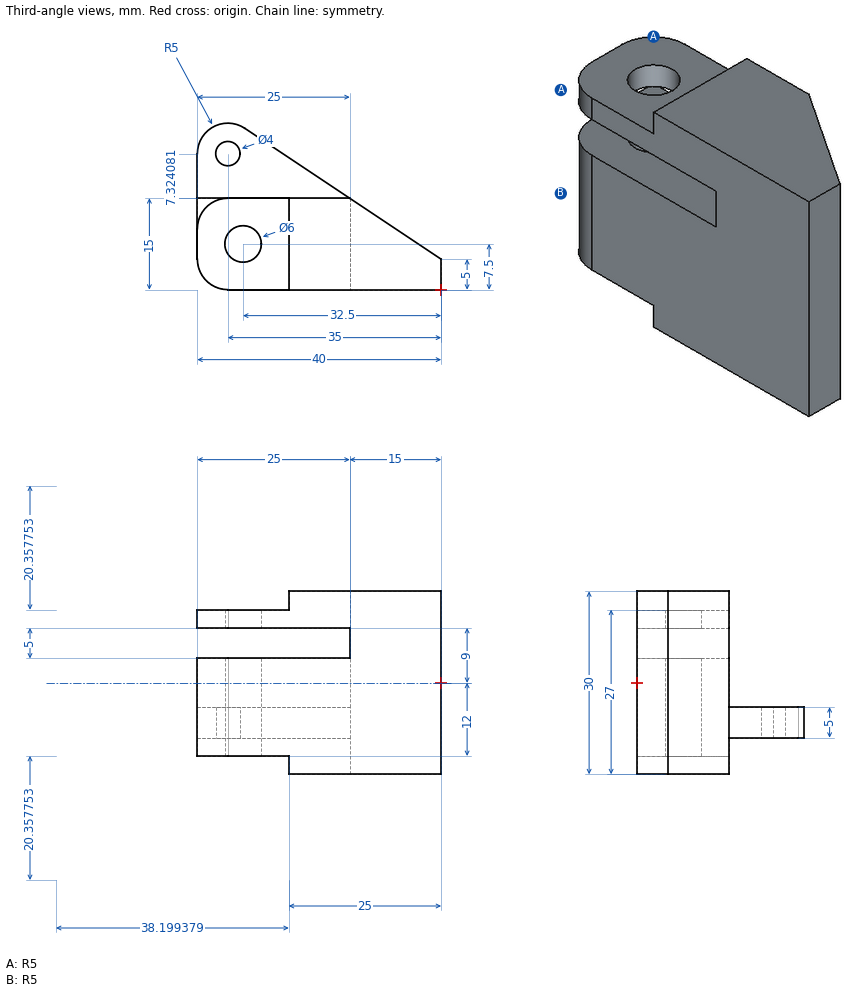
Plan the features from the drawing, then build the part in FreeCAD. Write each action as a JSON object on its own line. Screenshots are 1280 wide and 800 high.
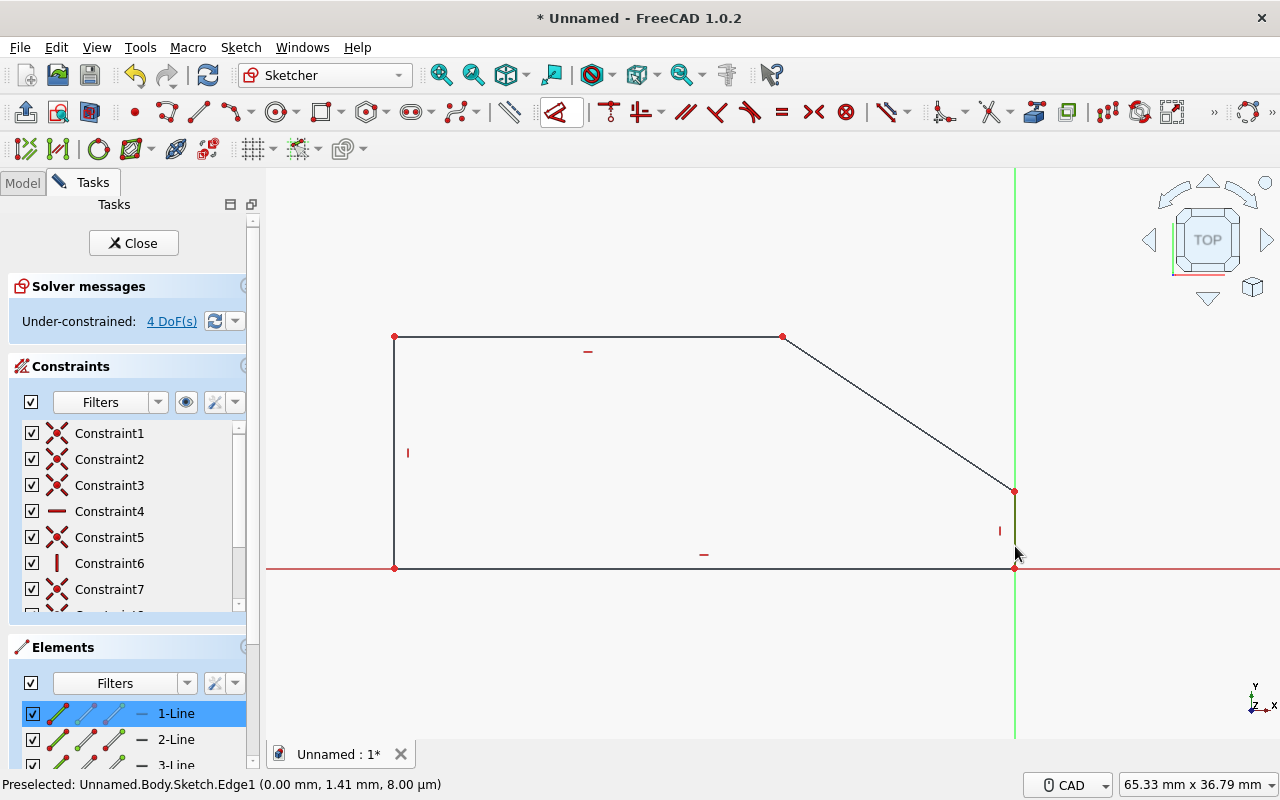
{"action": "key", "text": "i"}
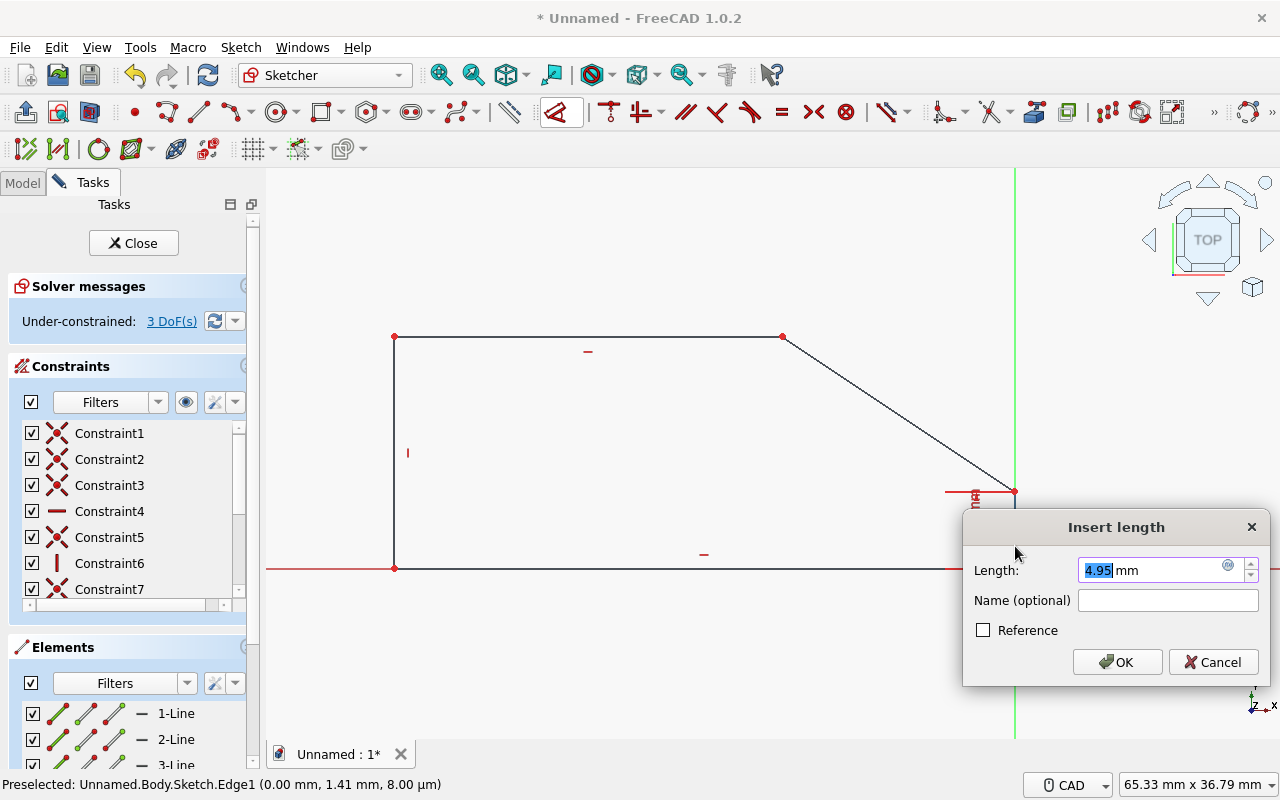
{"action": "type", "text": "5"}
{"action": "key", "text": "Return"}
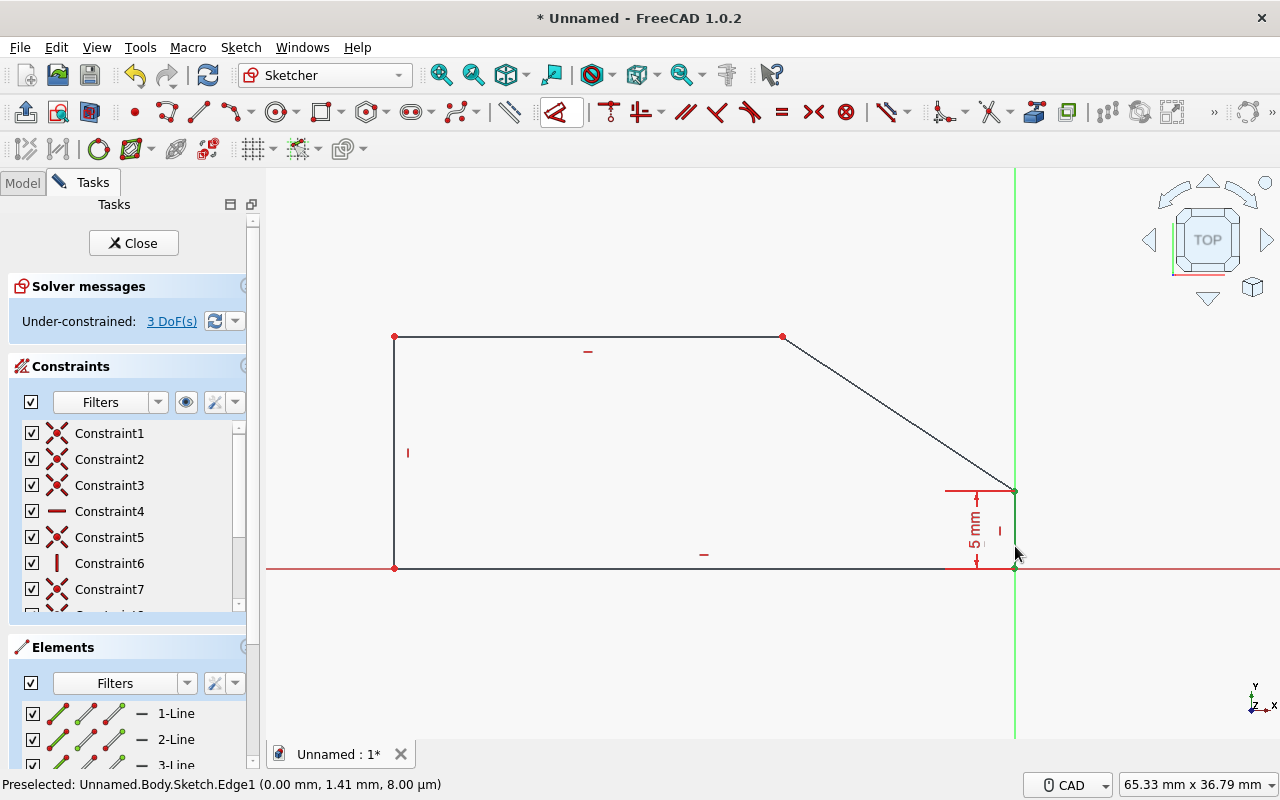
{"action": "left_click", "coordinate": [666, 337]}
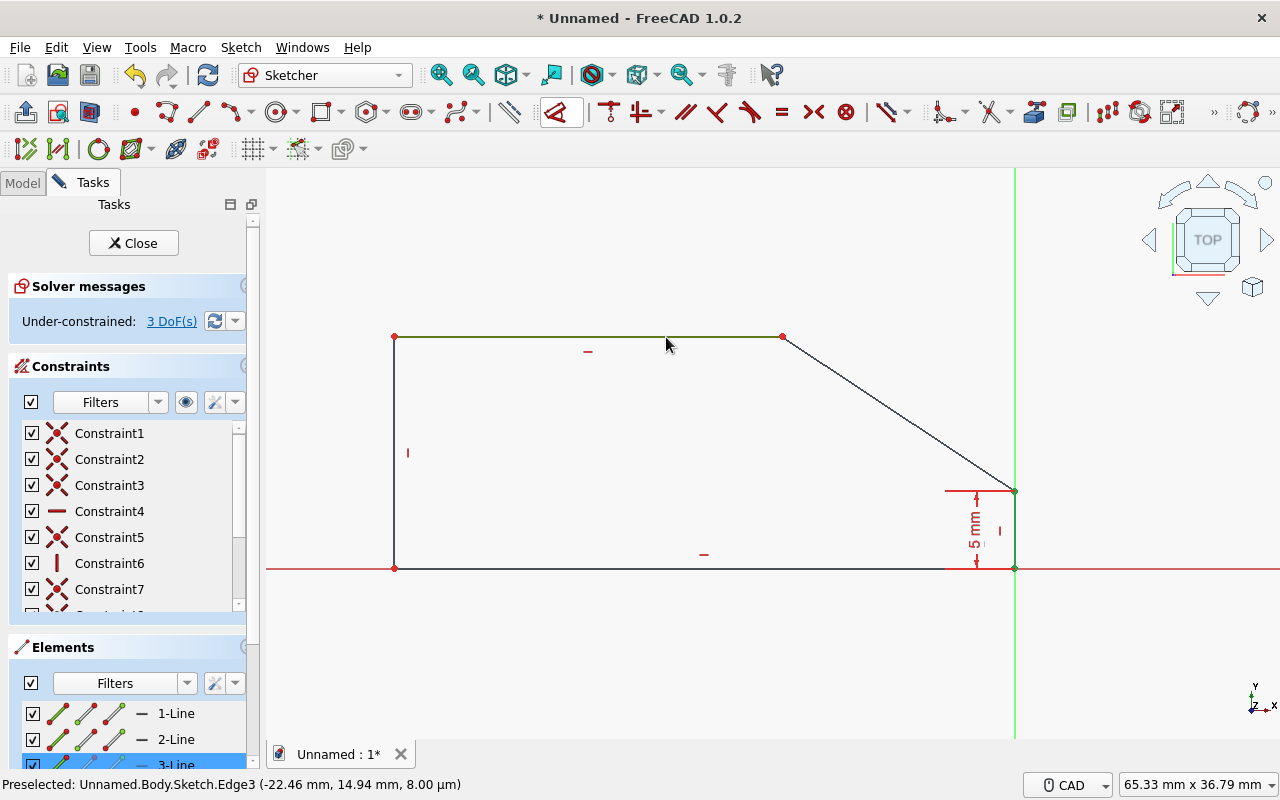
{"action": "key", "text": "l"}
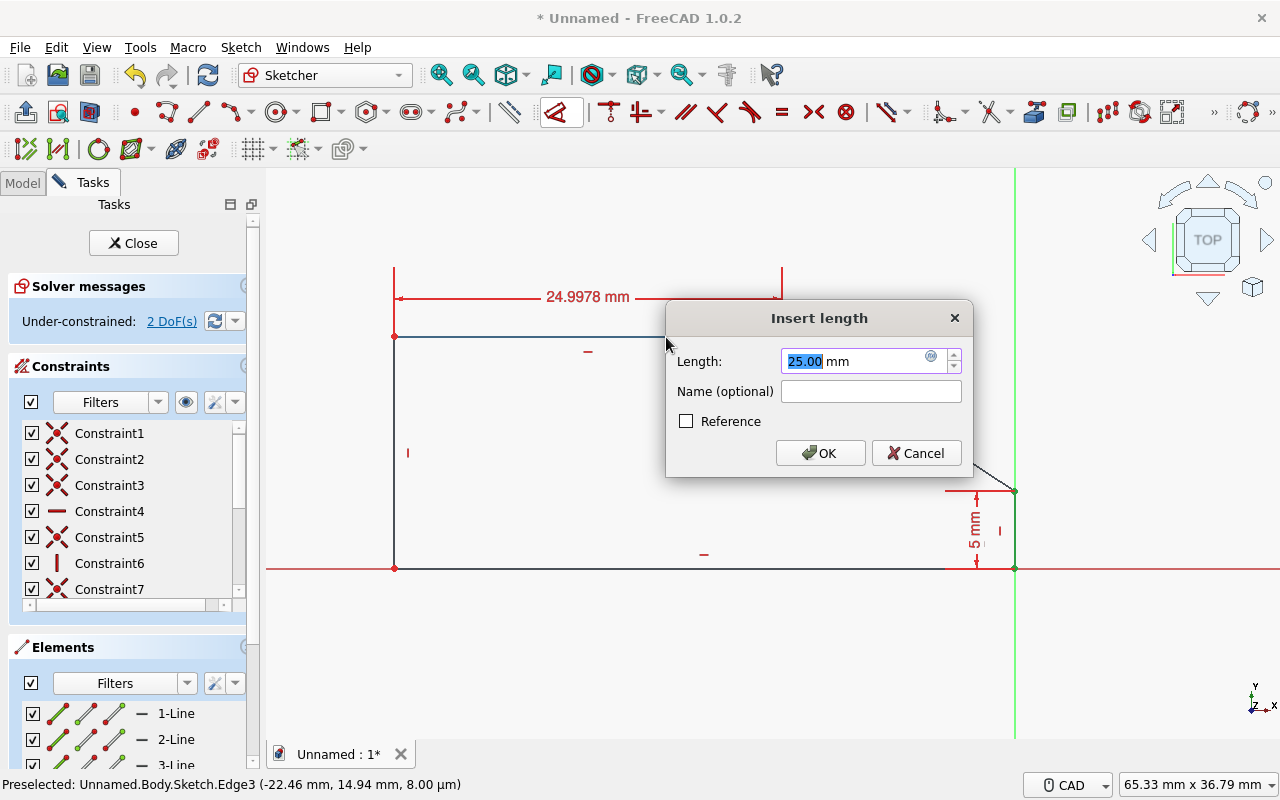
{"action": "type", "text": "25"}
{"action": "key", "text": "Return"}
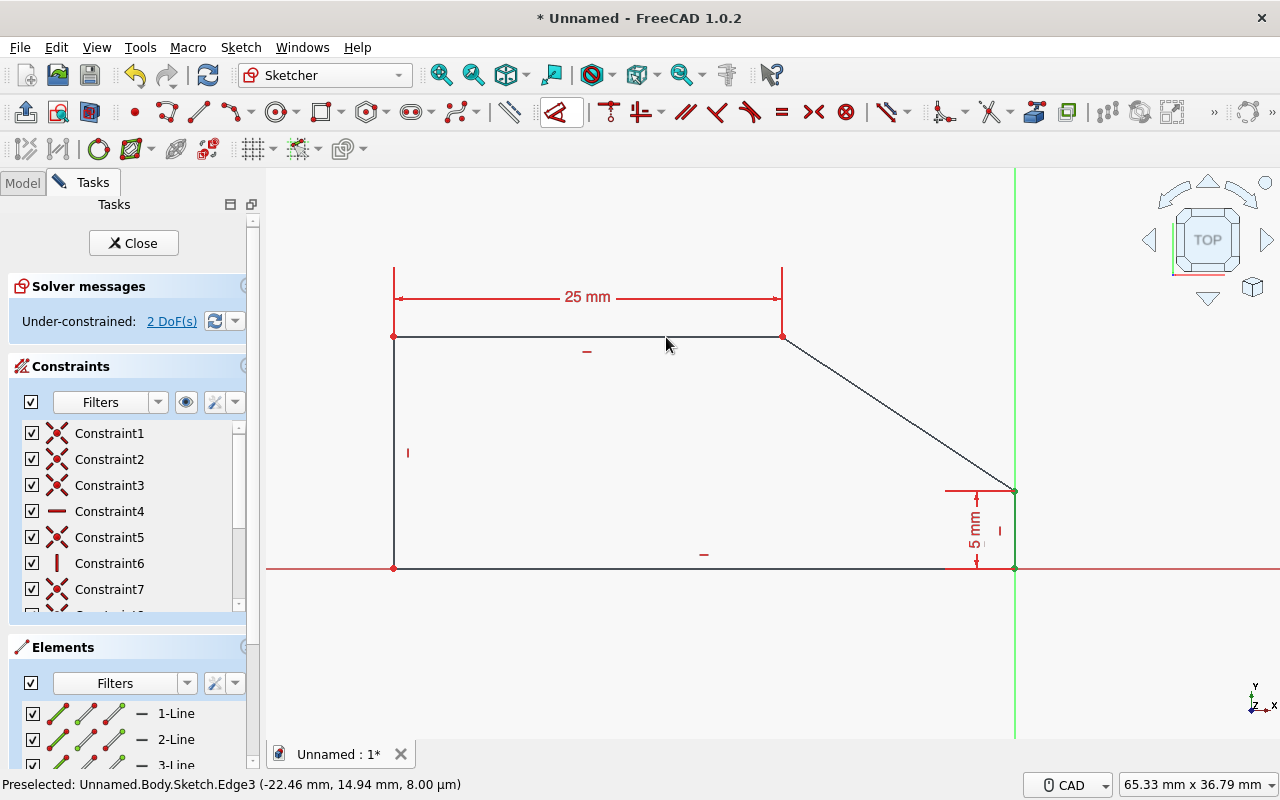
{"action": "left_click", "coordinate": [394, 407]}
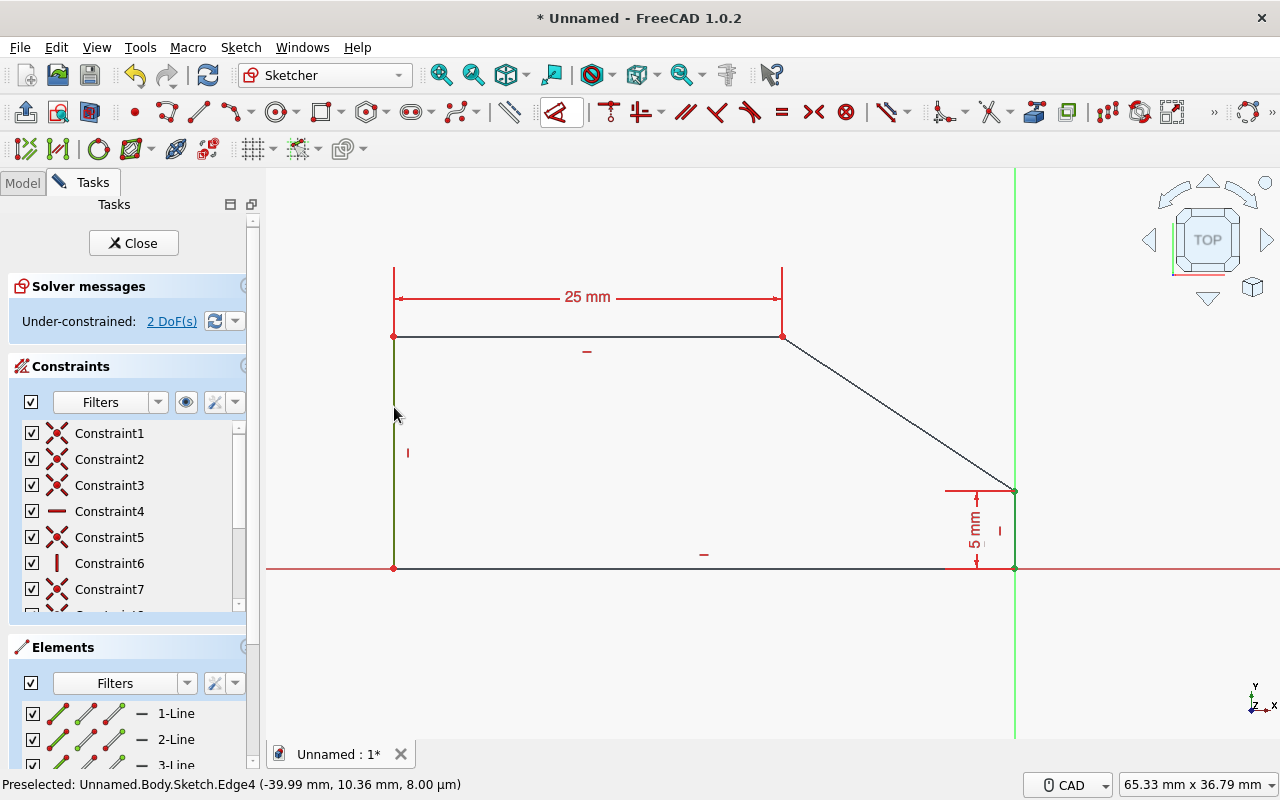
{"action": "left_click", "coordinate": [578, 112]}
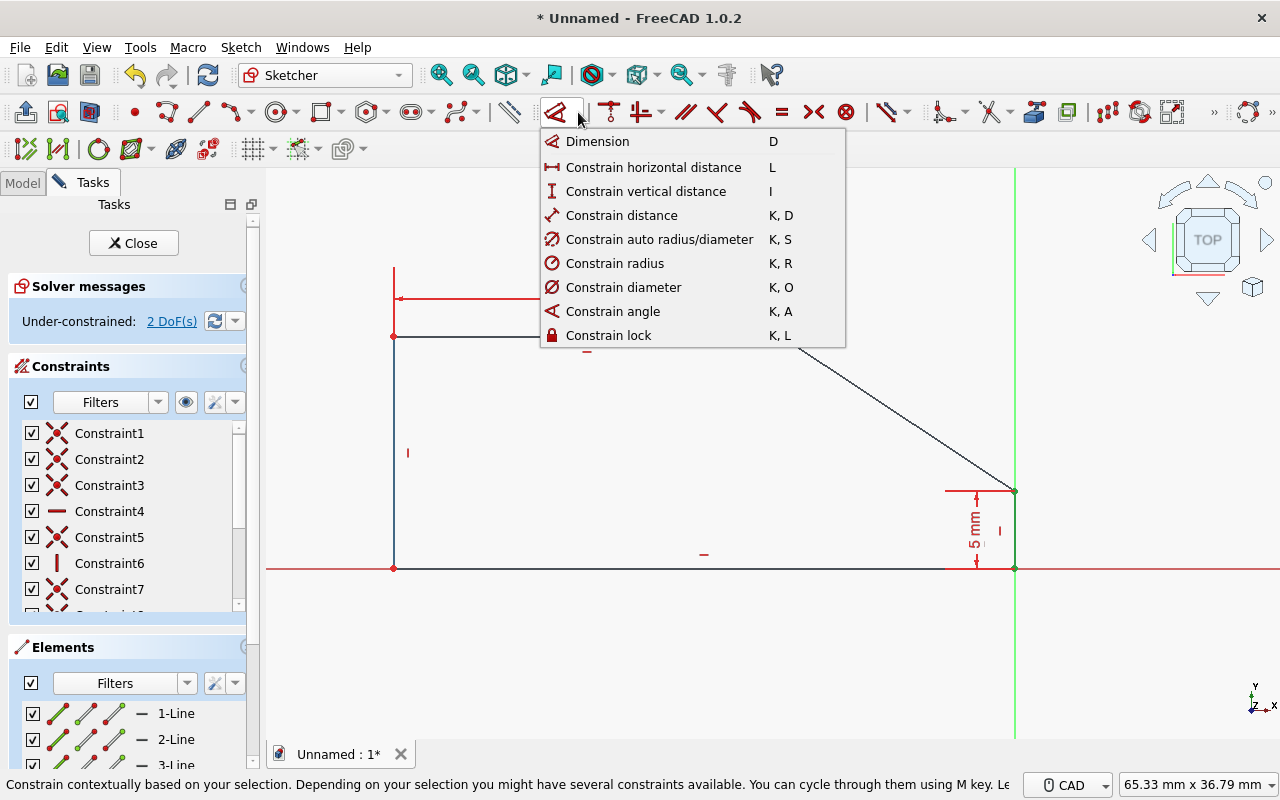
{"action": "left_click", "coordinate": [693, 191]}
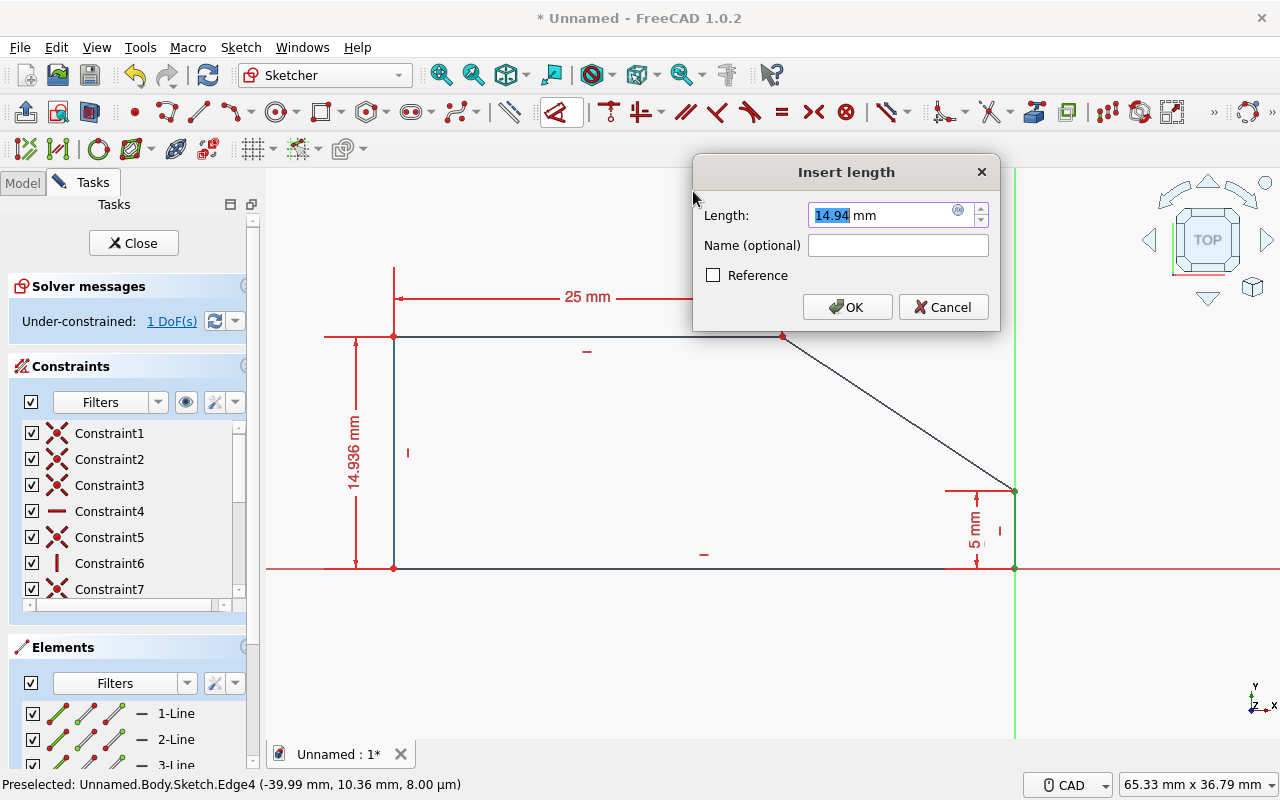
{"action": "type", "text": "15"}
{"action": "key", "text": "Return"}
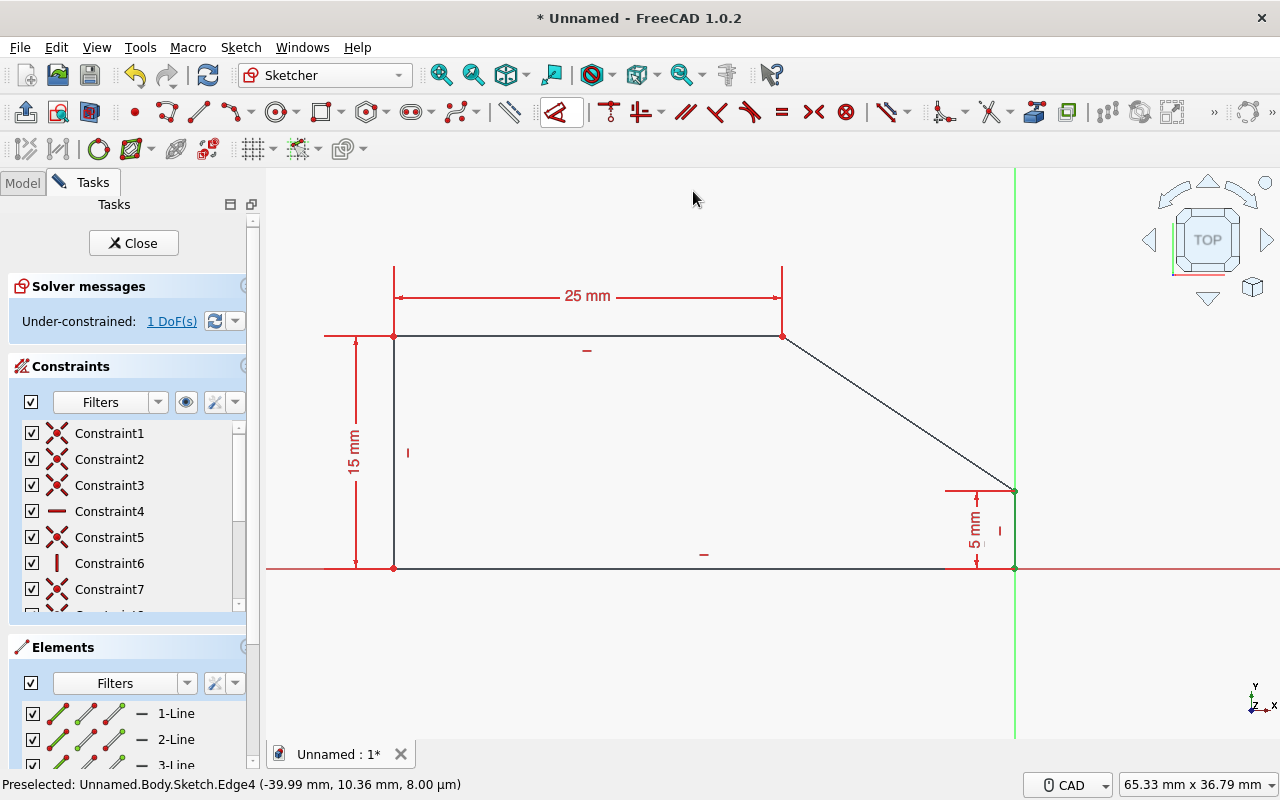
{"action": "left_click", "coordinate": [580, 569]}